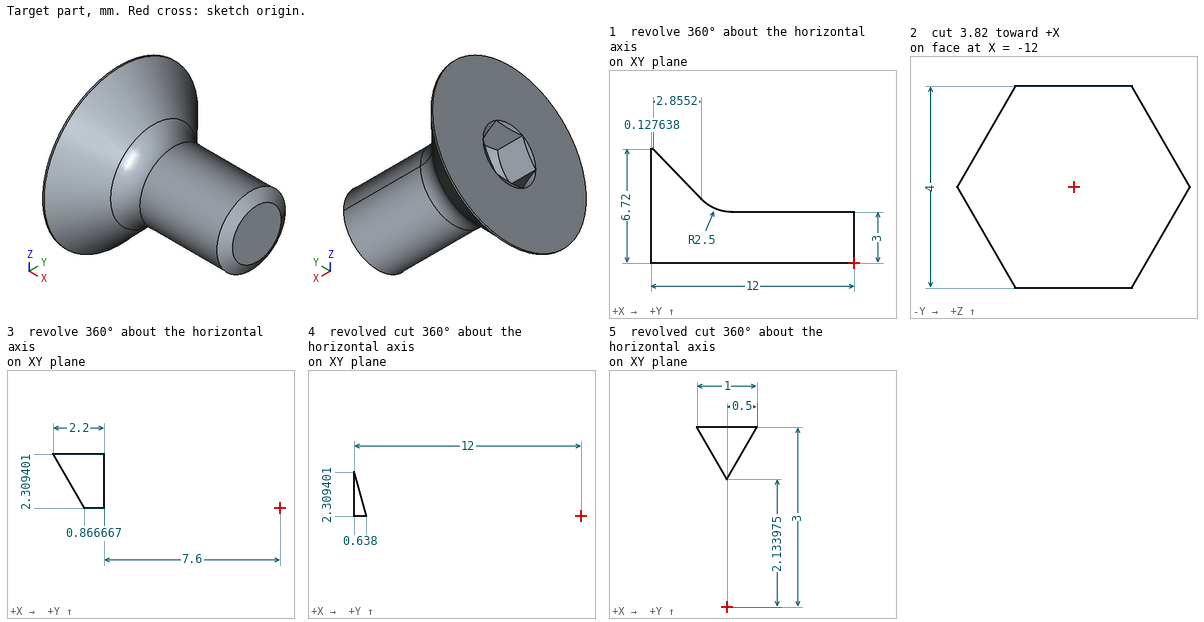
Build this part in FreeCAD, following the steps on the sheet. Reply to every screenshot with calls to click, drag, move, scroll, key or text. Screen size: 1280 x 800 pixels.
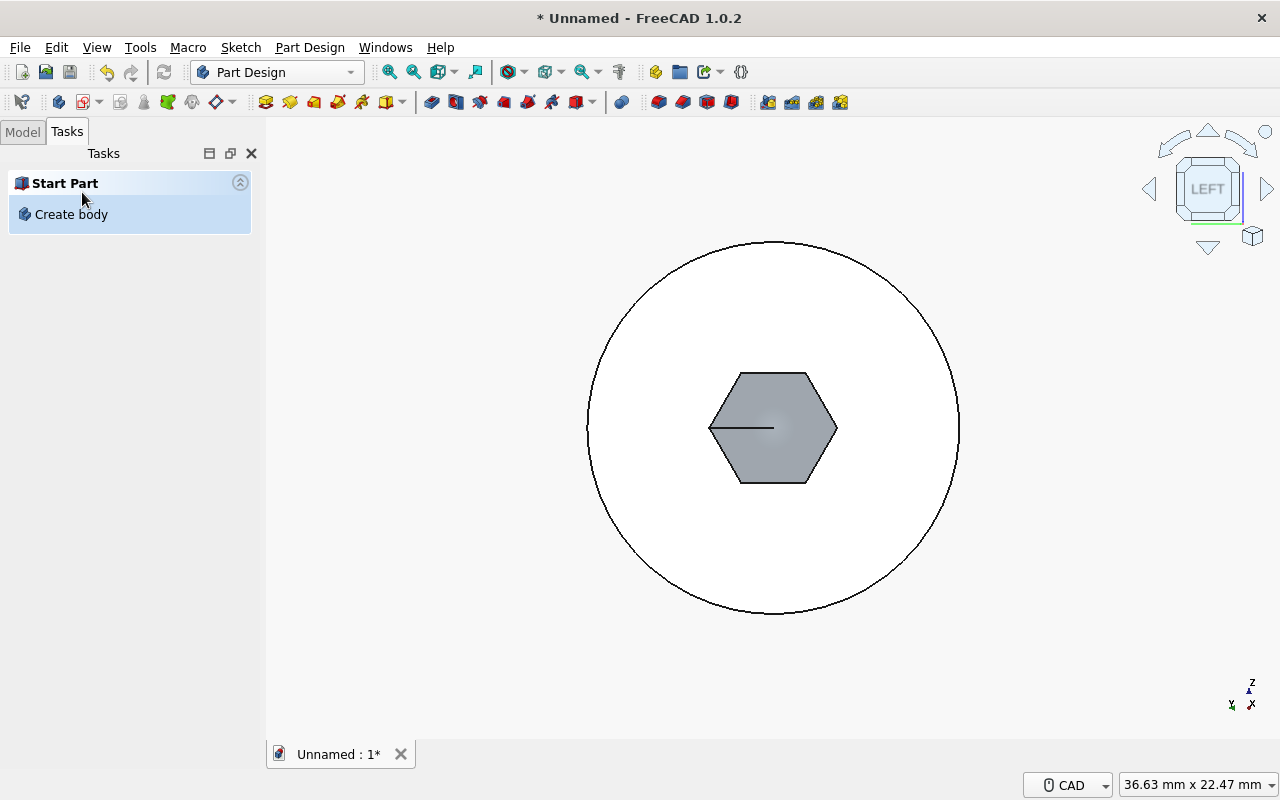
click(84, 102)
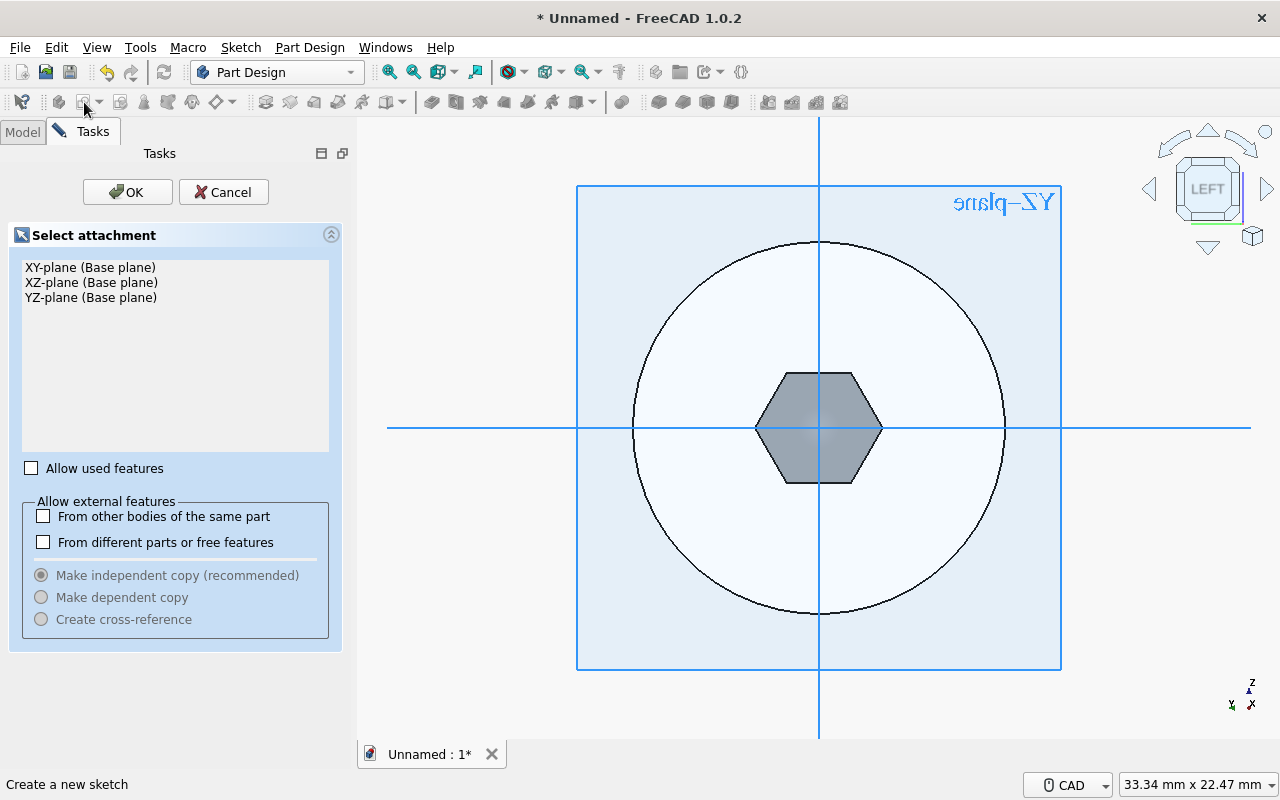
click(82, 268)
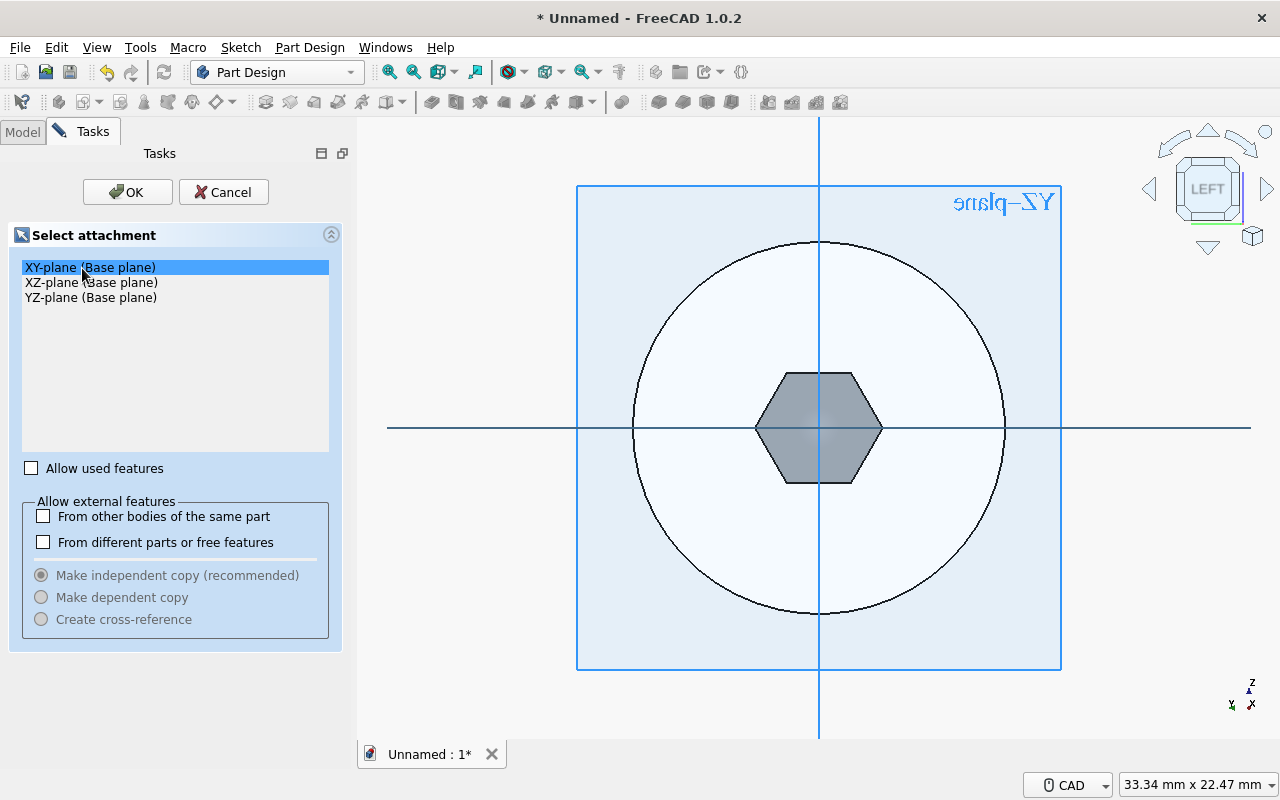
click(128, 192)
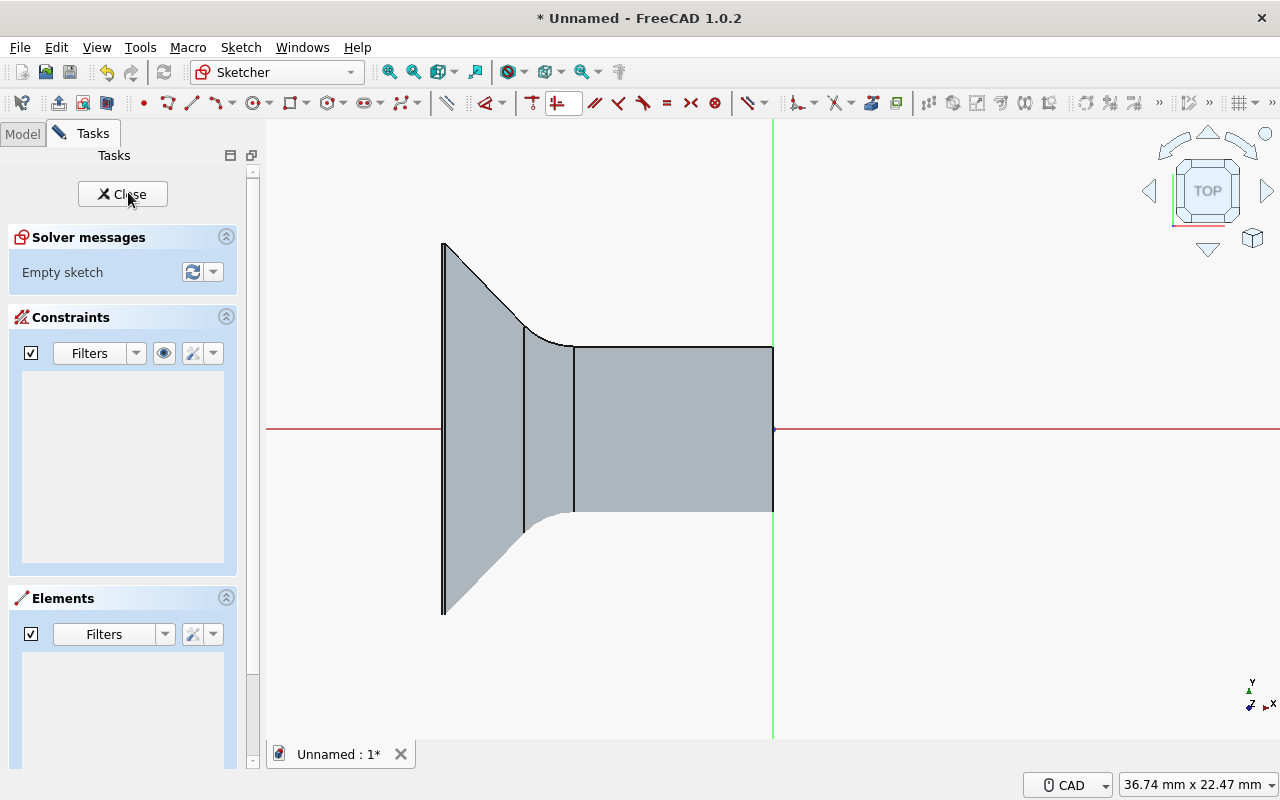
key(q)
key(s)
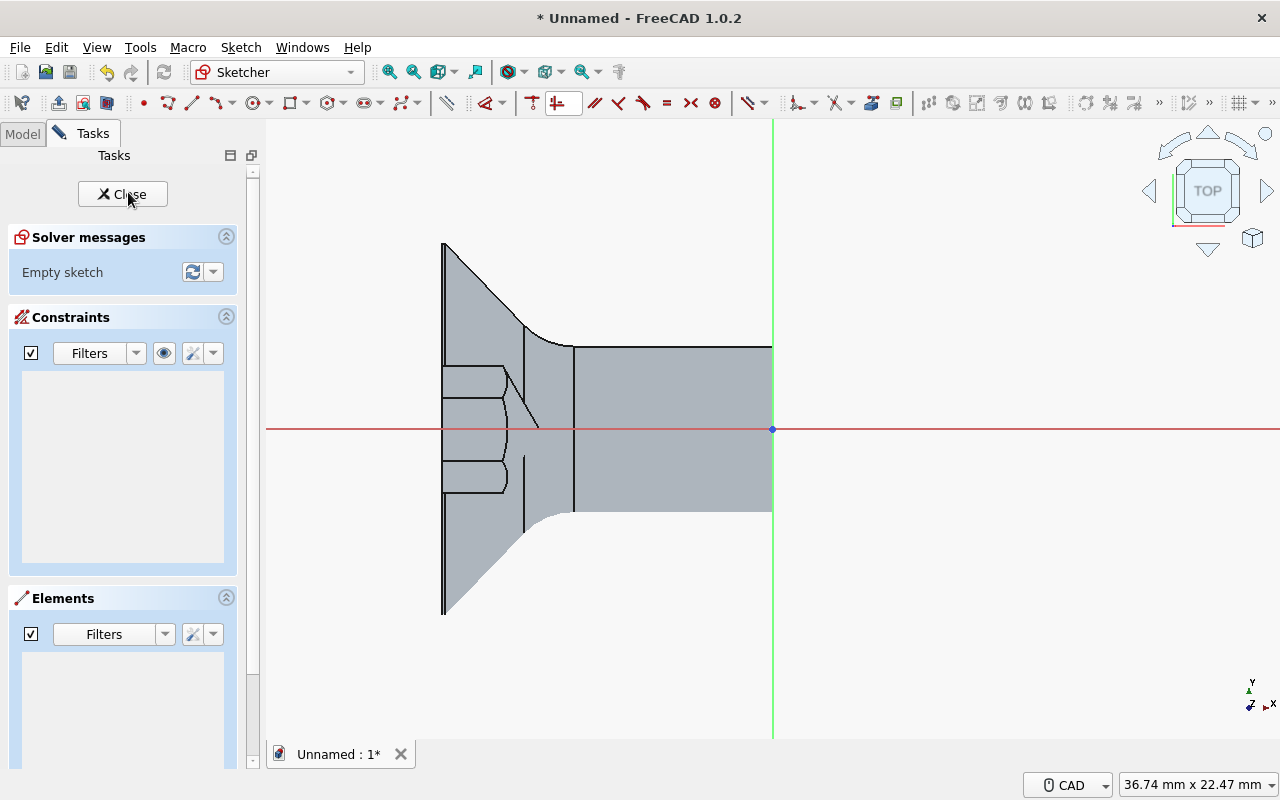
scroll(400, 391, up, 9)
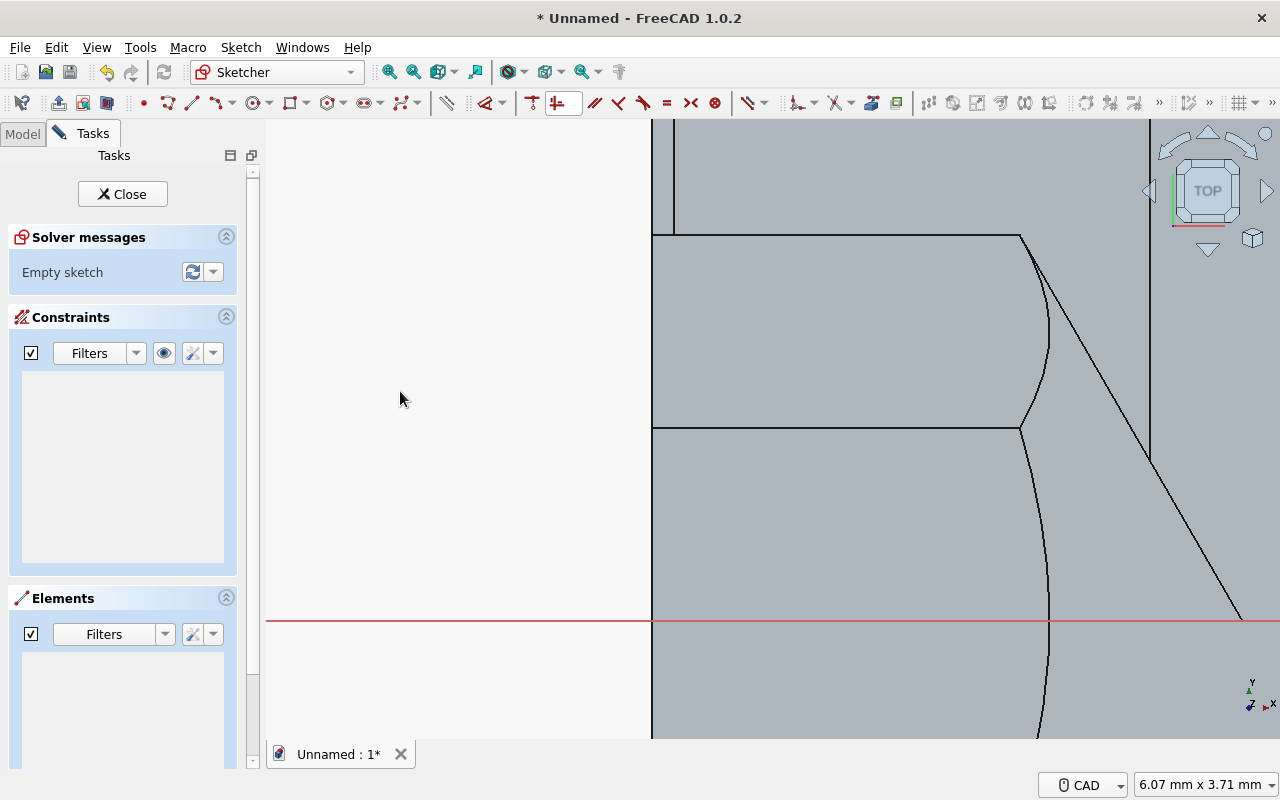
key(g)
key(m)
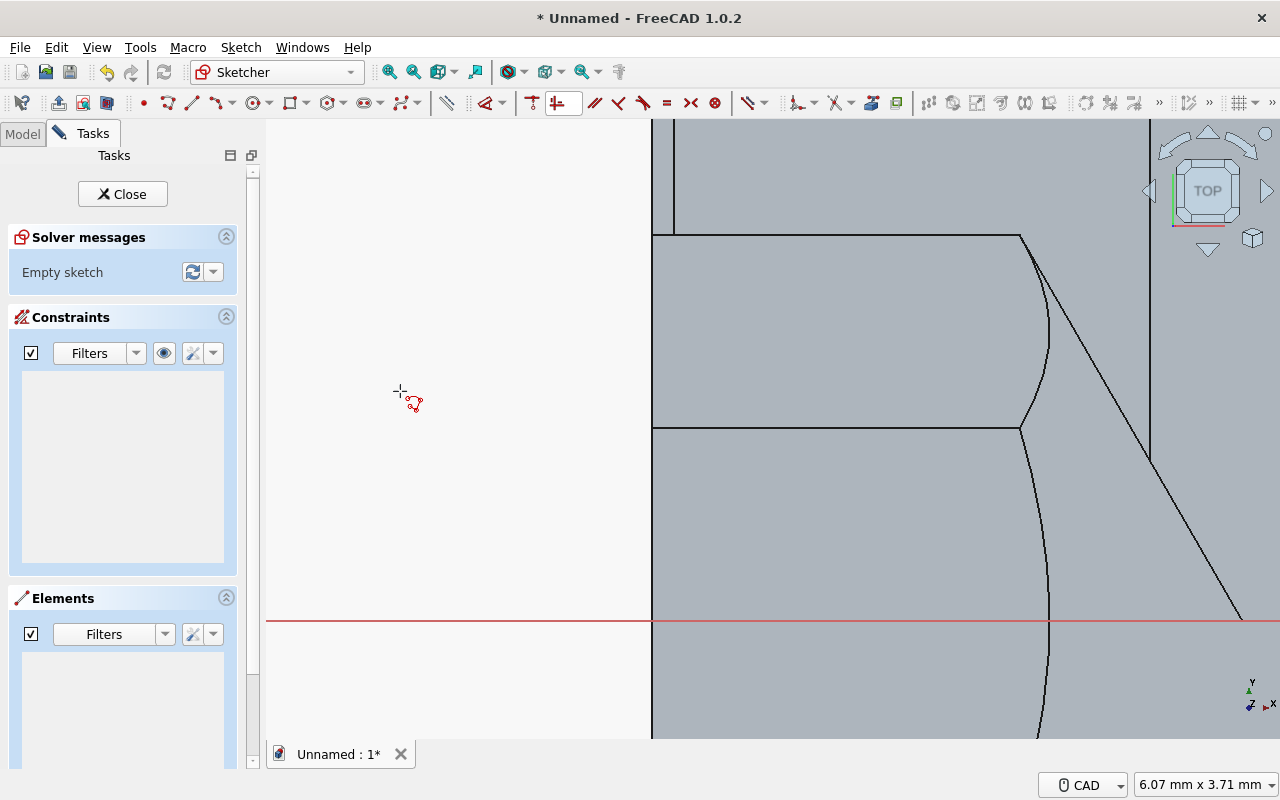
click(759, 621)
click(652, 235)
click(652, 612)
click(759, 621)
key(Escape)
key(Escape)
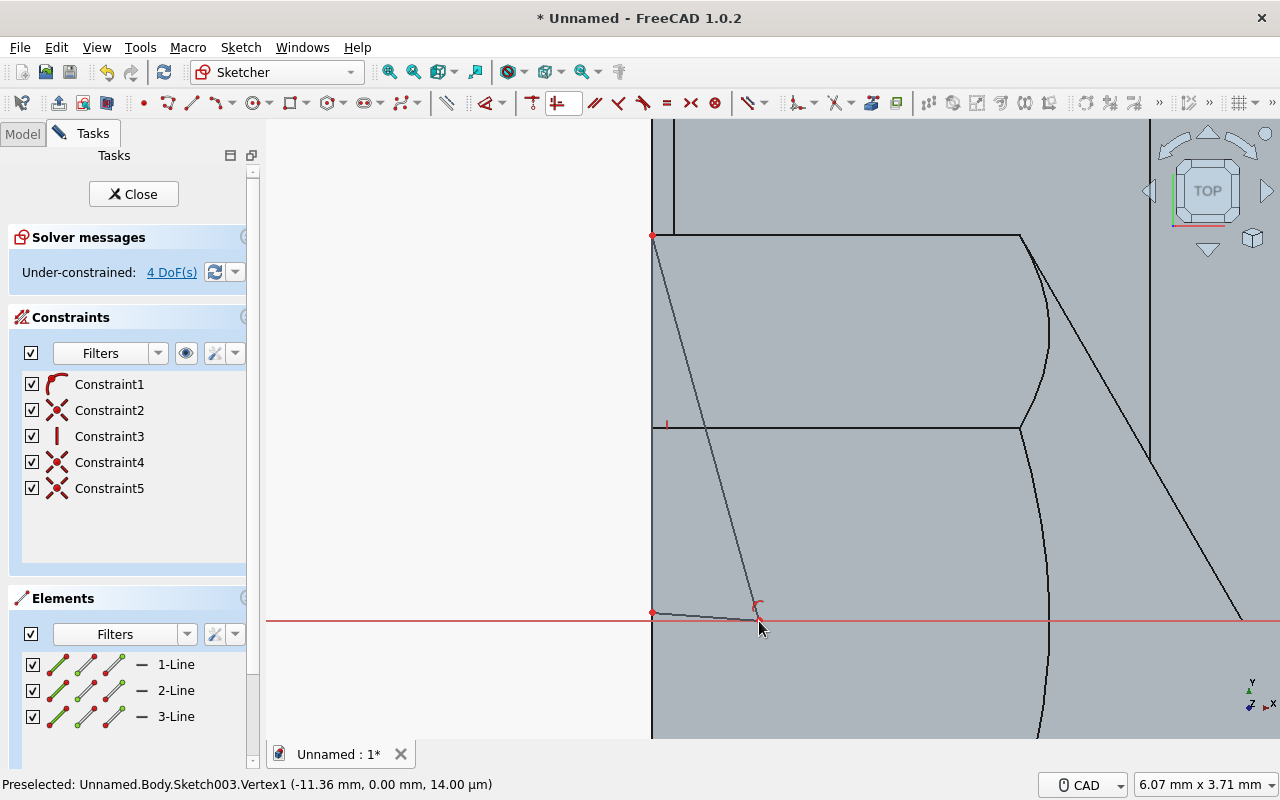
click(727, 619)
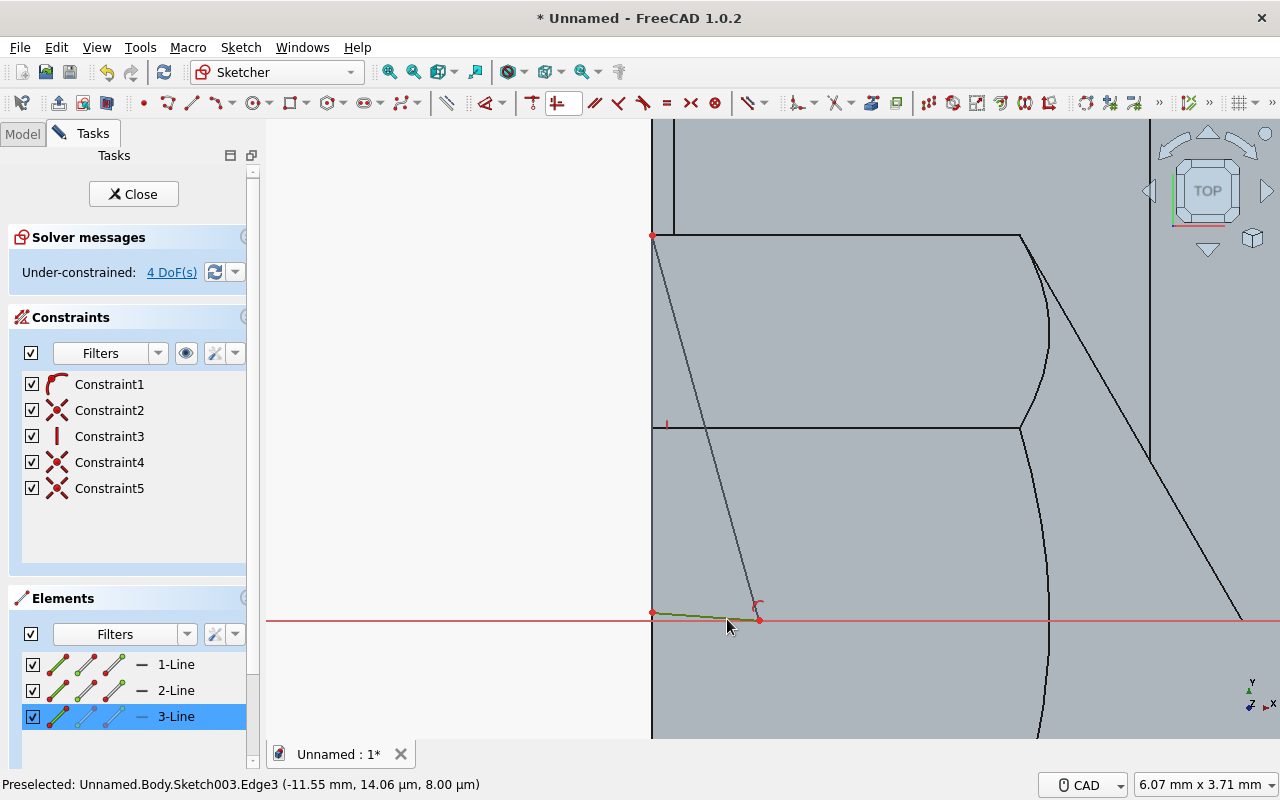
key(h)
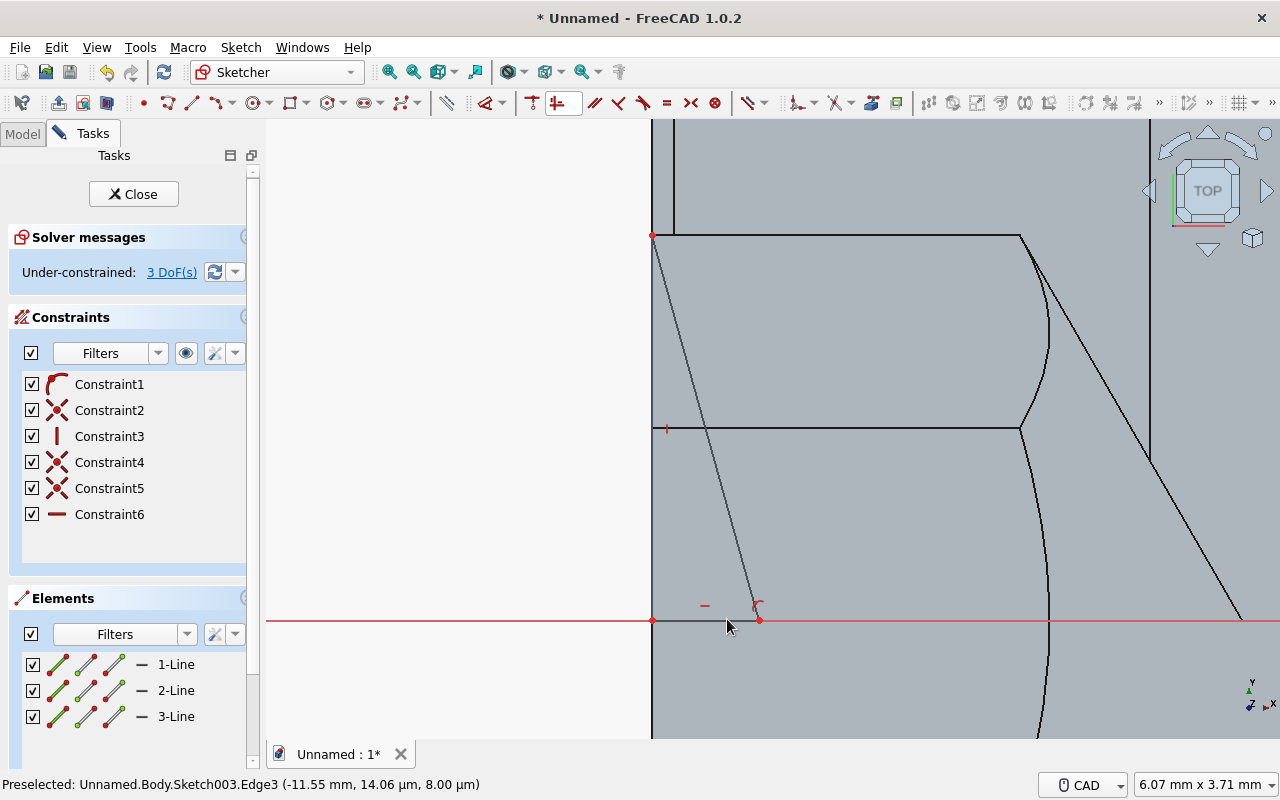
key(d)